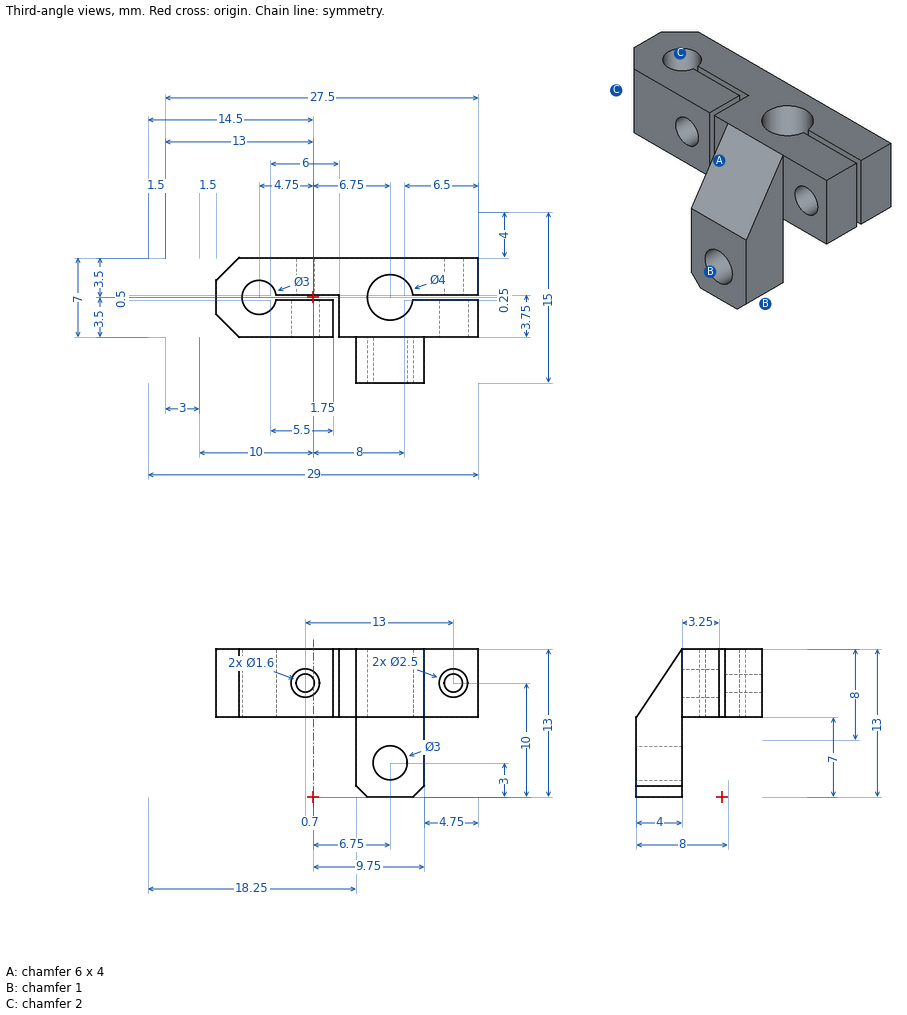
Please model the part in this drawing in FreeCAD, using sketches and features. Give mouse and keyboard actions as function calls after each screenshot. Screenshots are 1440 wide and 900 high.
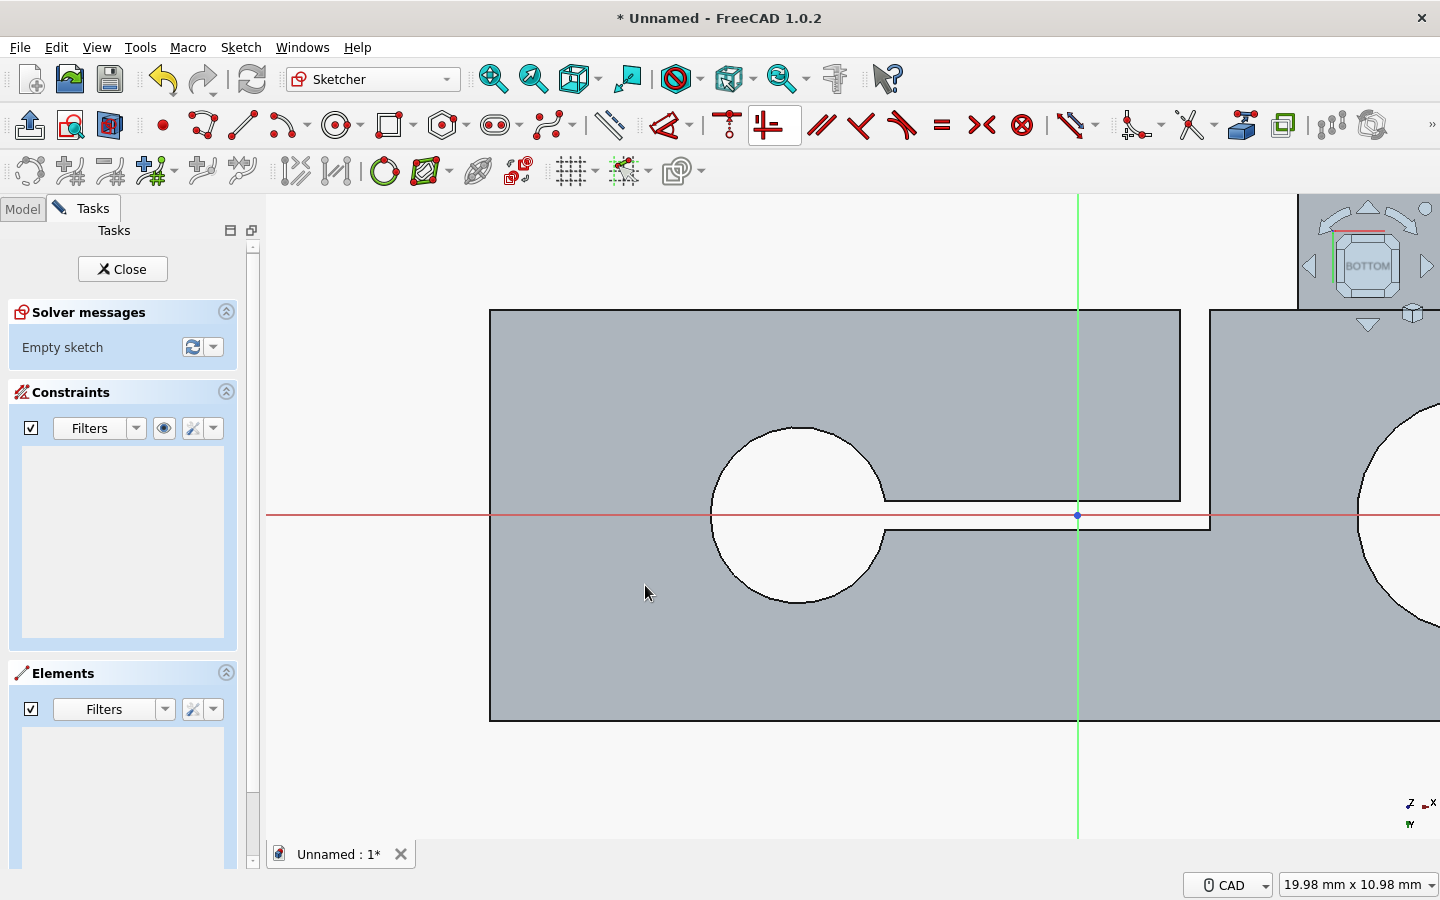
click(390, 126)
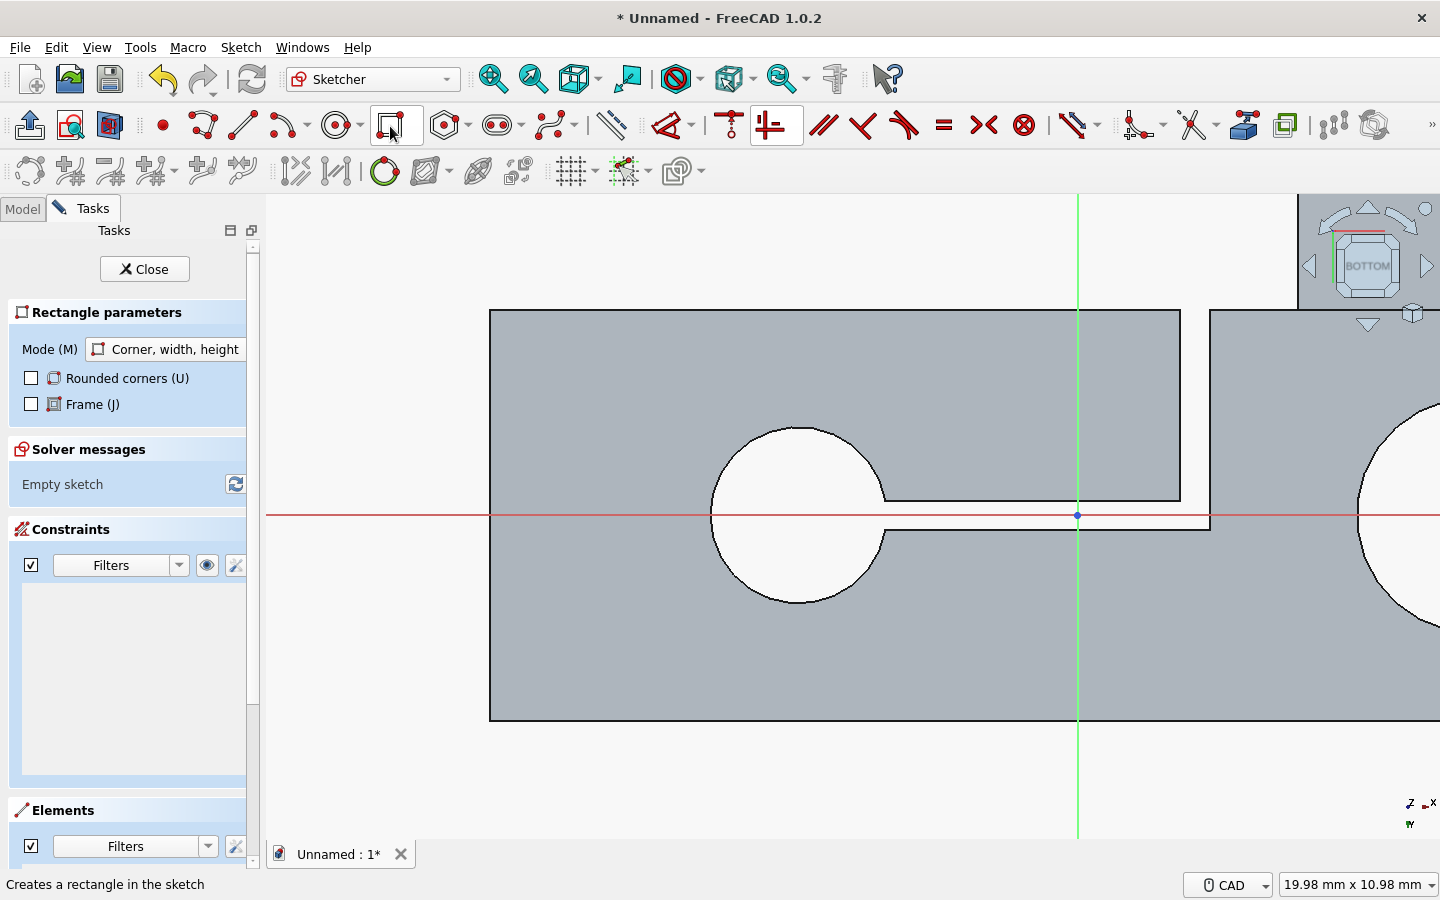
click(490, 310)
move(578, 721)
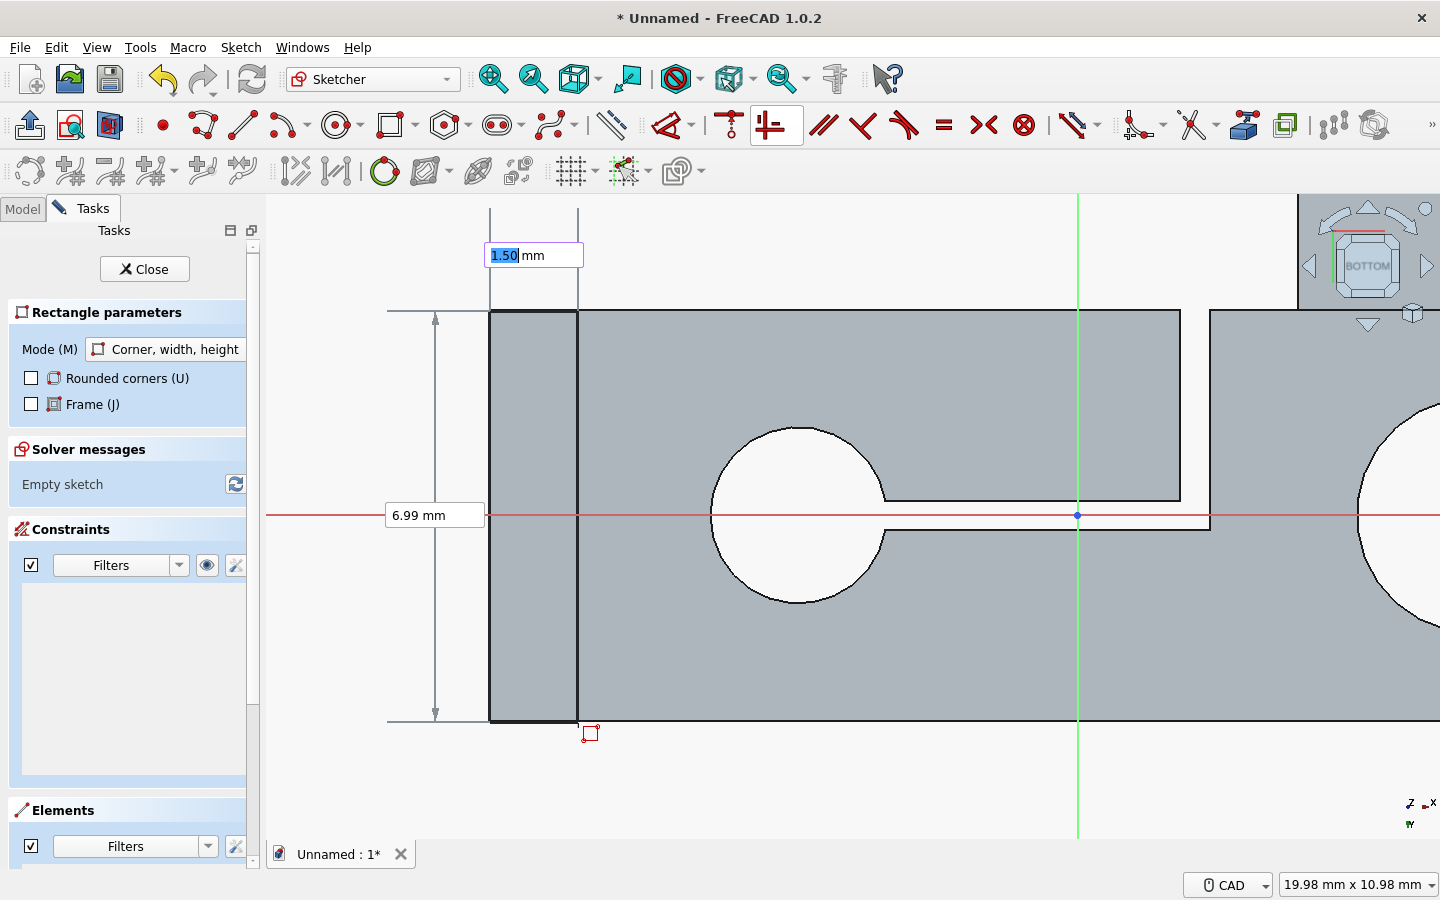
text(1.5)
key(Tab)
text(7)
key(Return)
key(Escape)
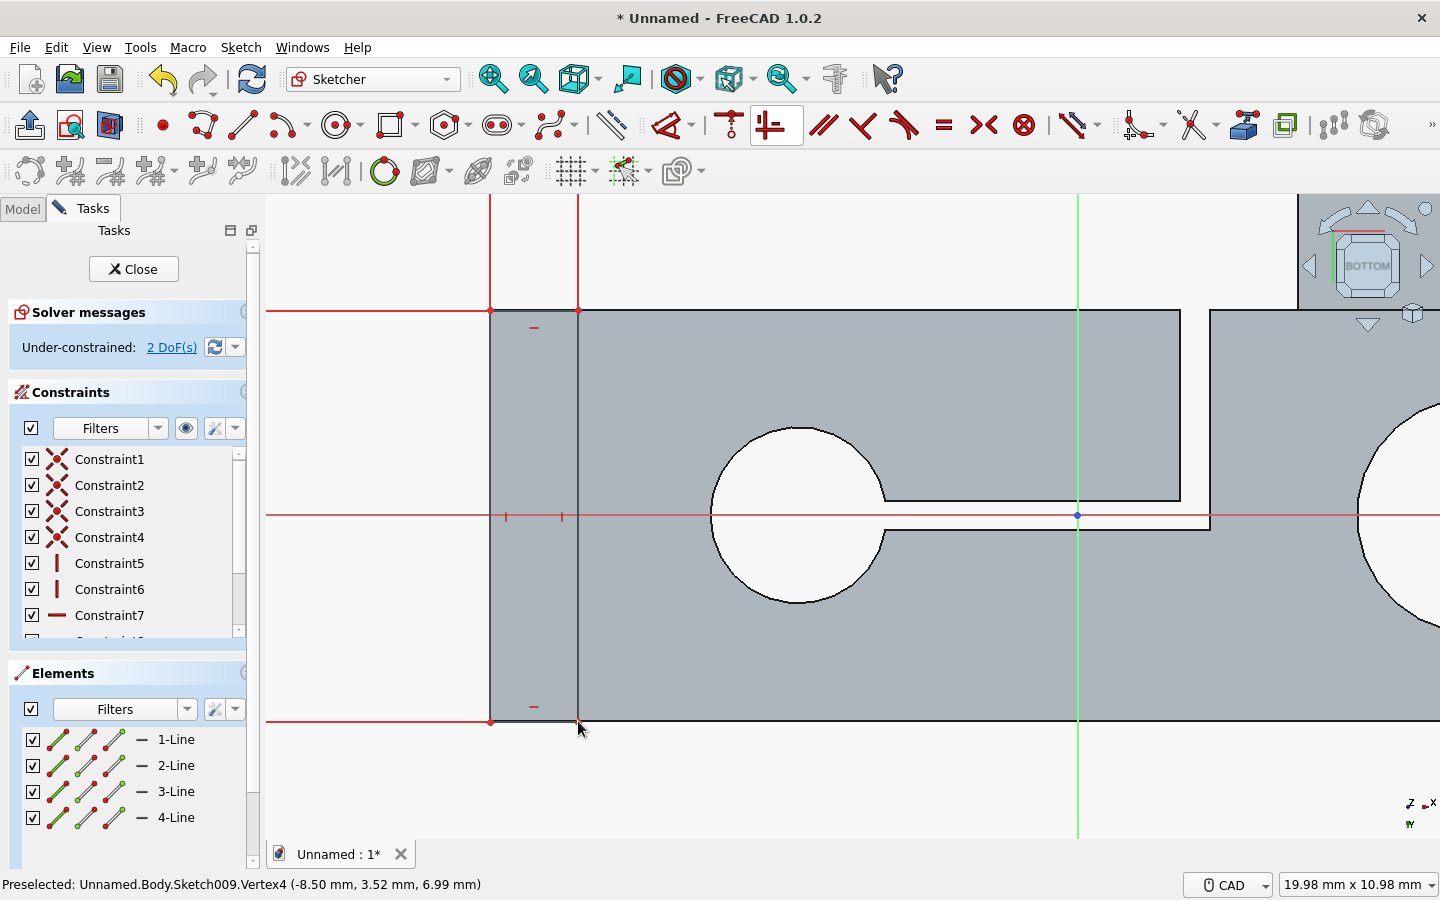
click(666, 126)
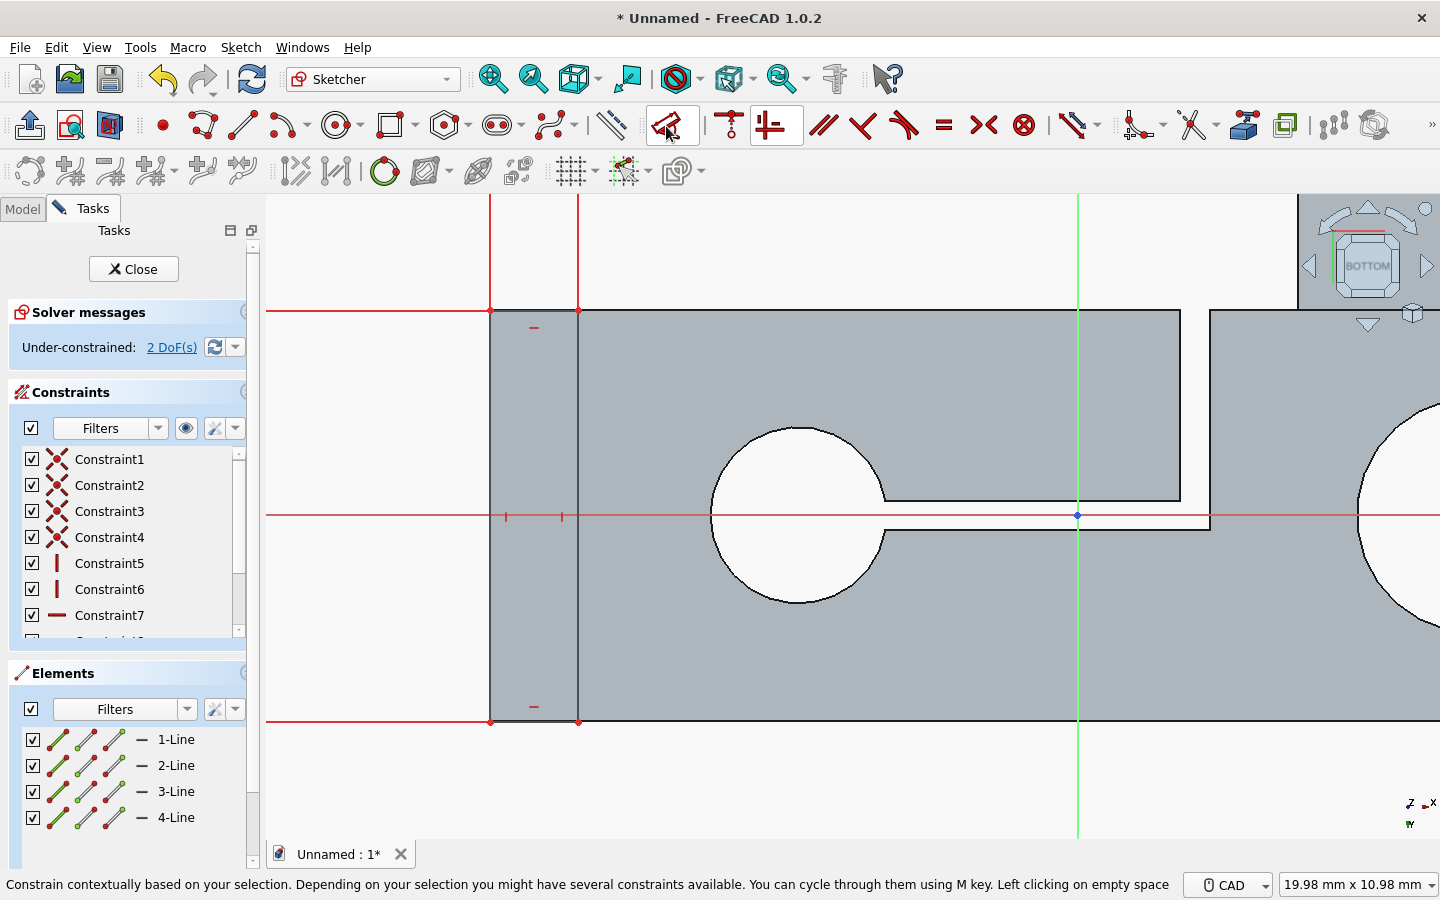
click(490, 311)
click(784, 277)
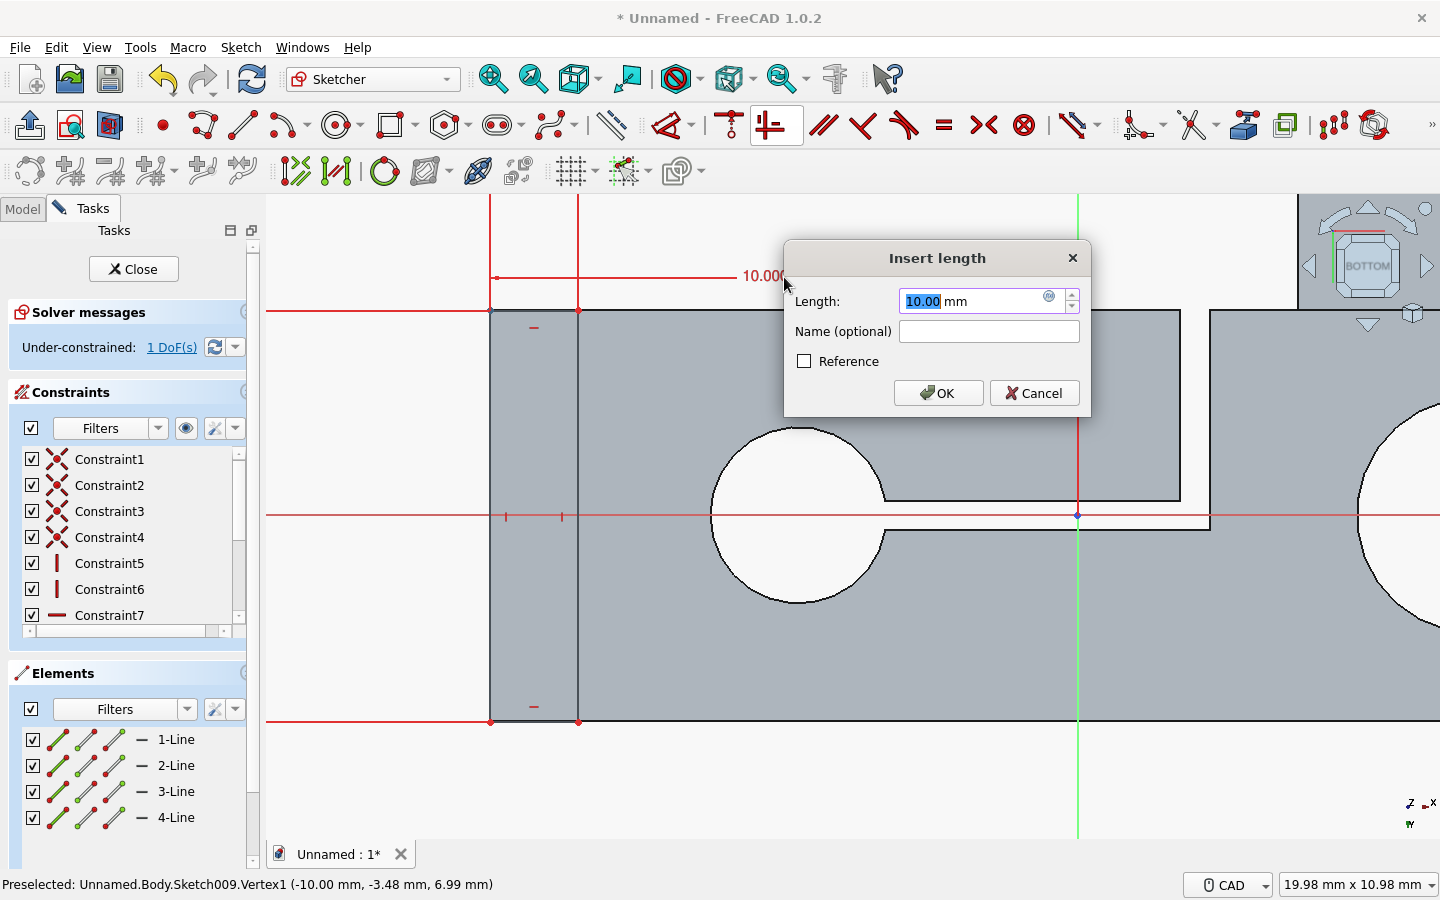
text(10)
key(Return)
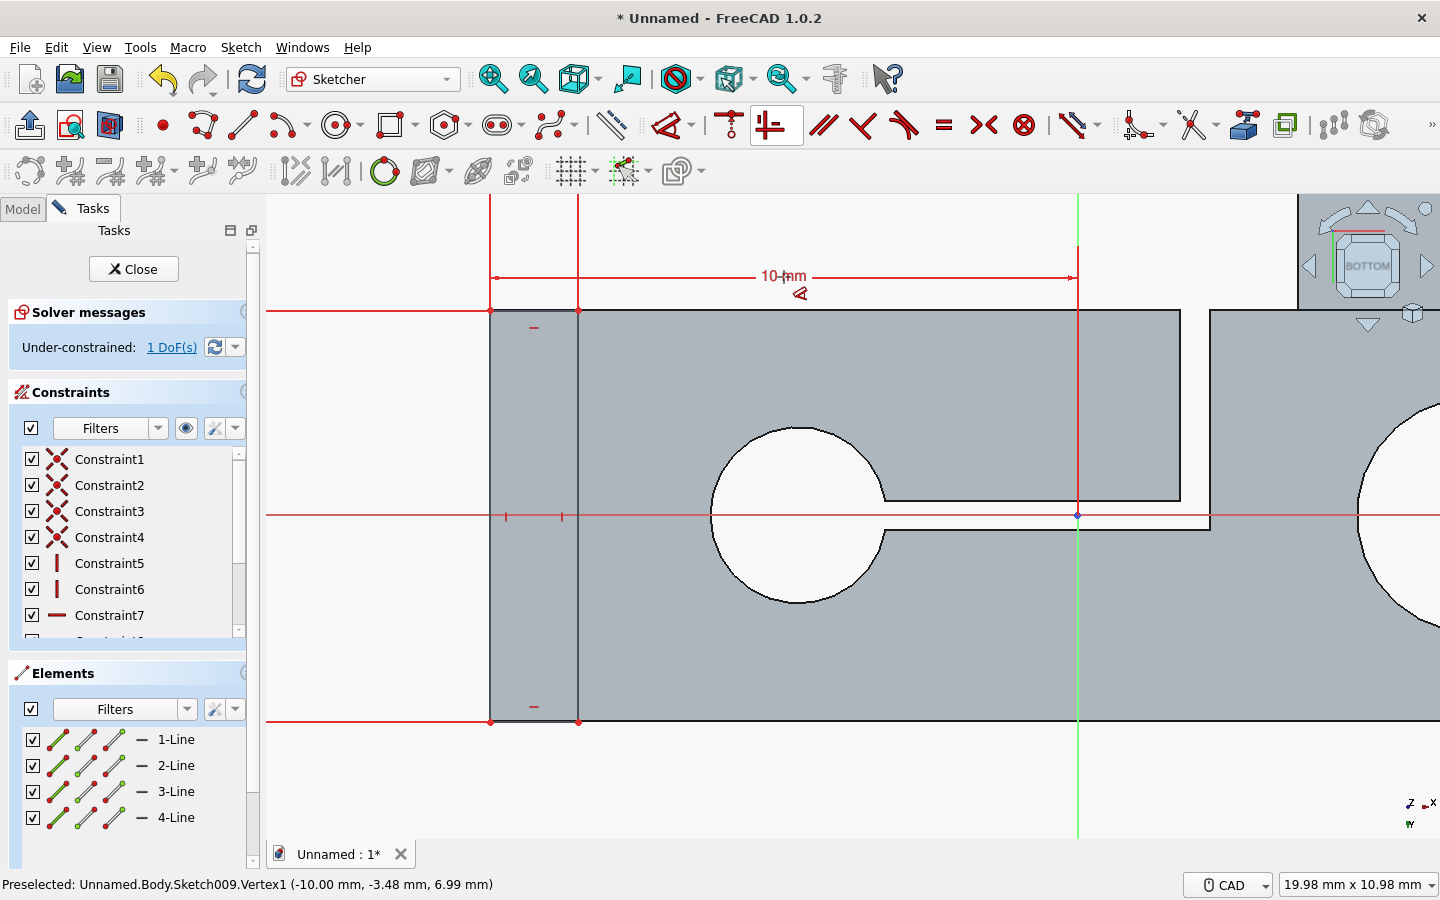
click(490, 311)
click(1112, 413)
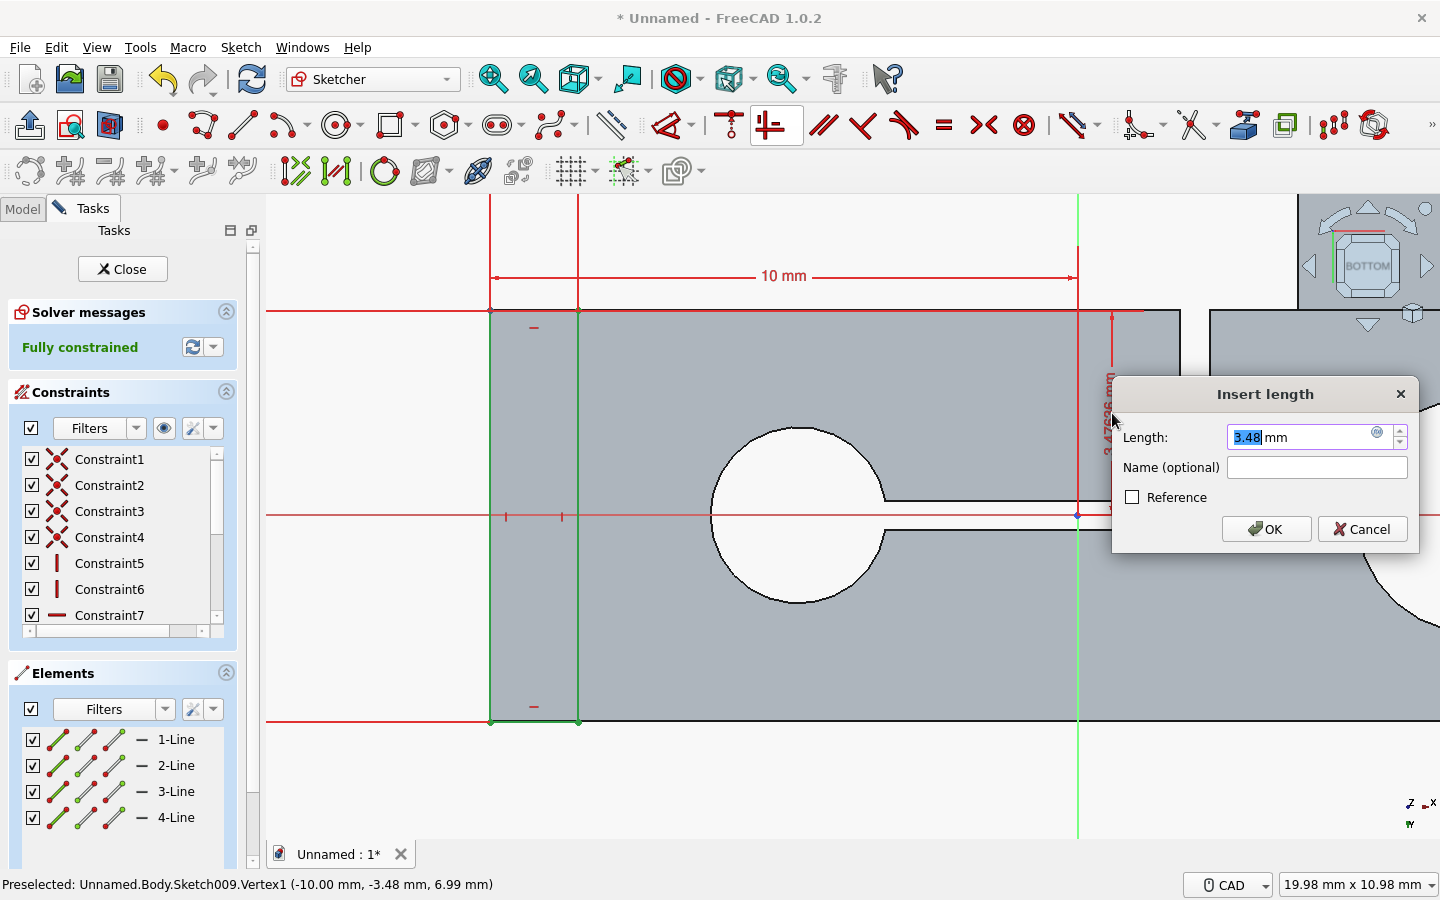
text(3.5)
key(Return)
key(Escape)